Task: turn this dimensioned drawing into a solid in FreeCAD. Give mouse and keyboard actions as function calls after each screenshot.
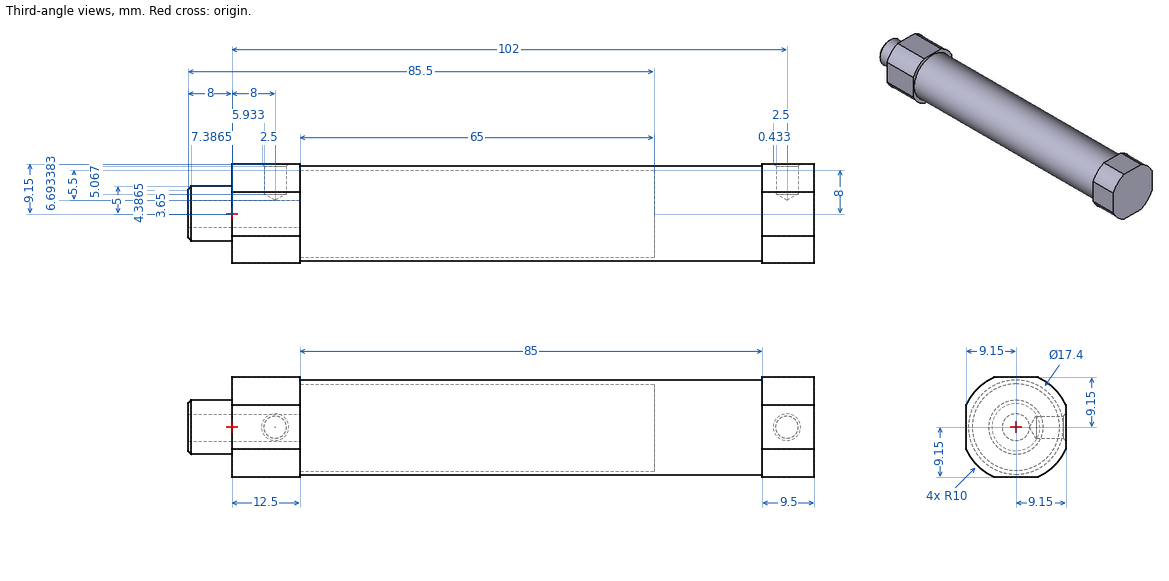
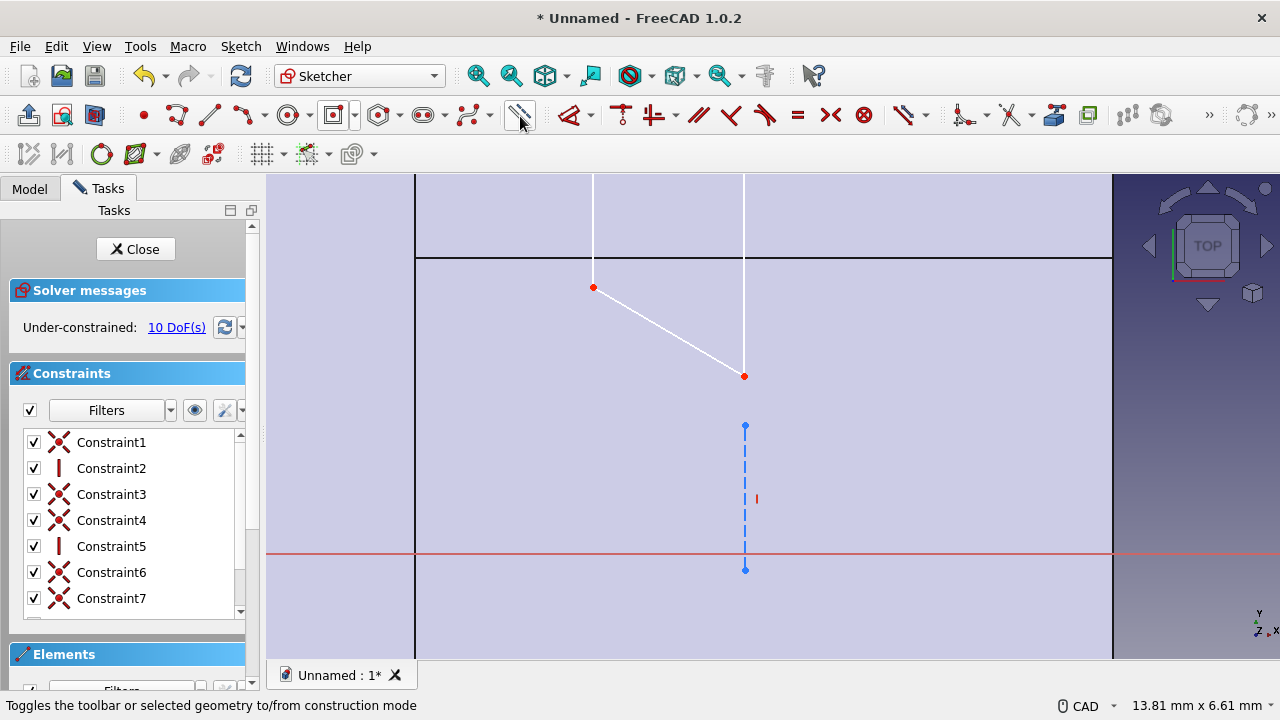
click(568, 116)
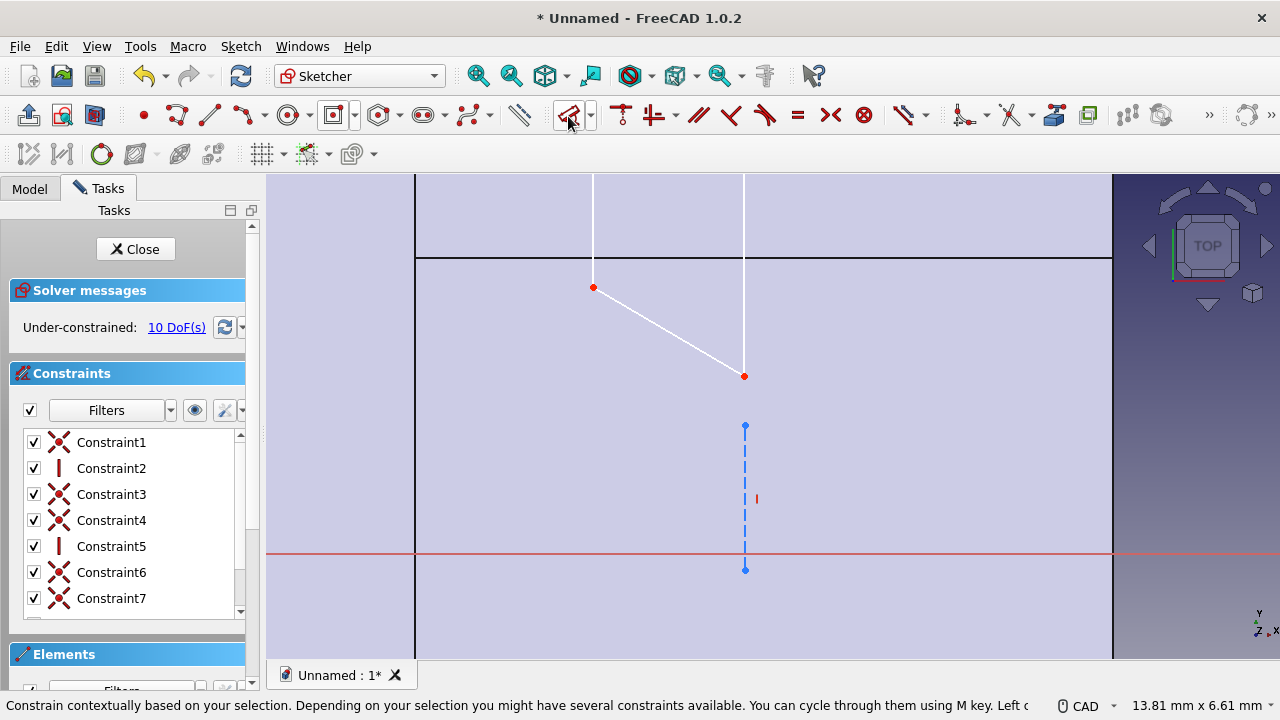
scroll(746, 572, down, 4)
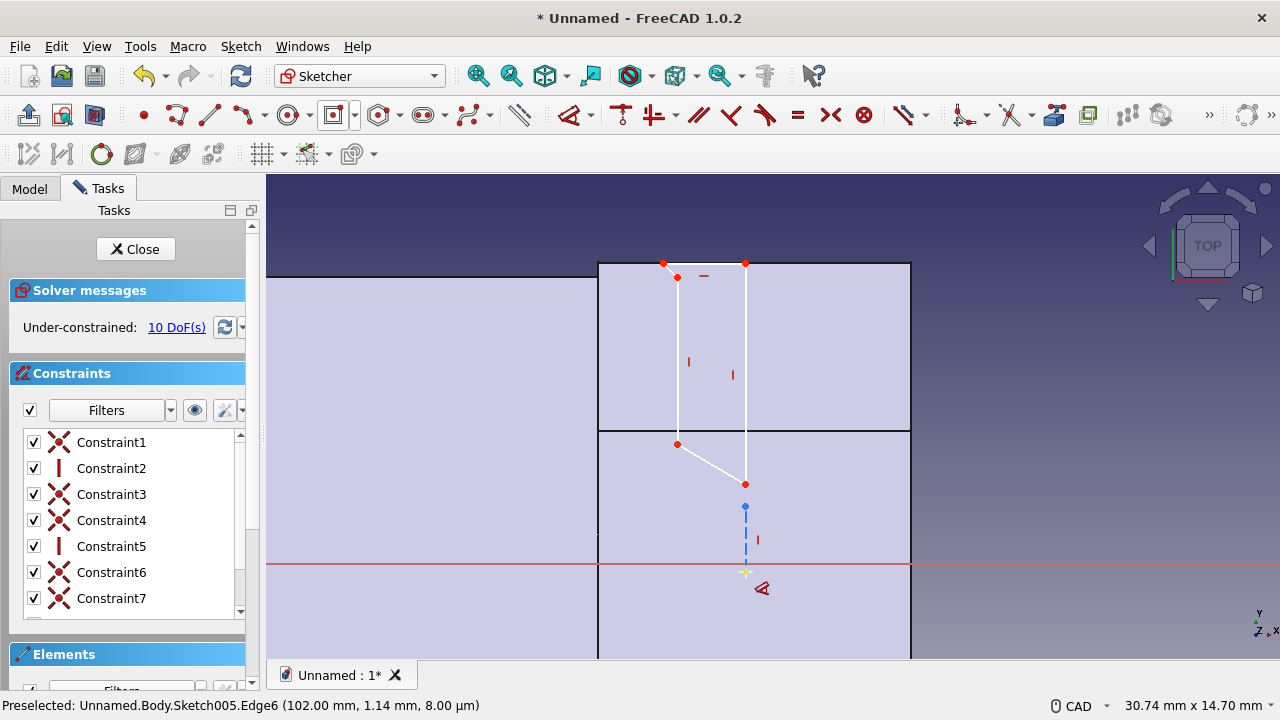
click(721, 264)
click(705, 230)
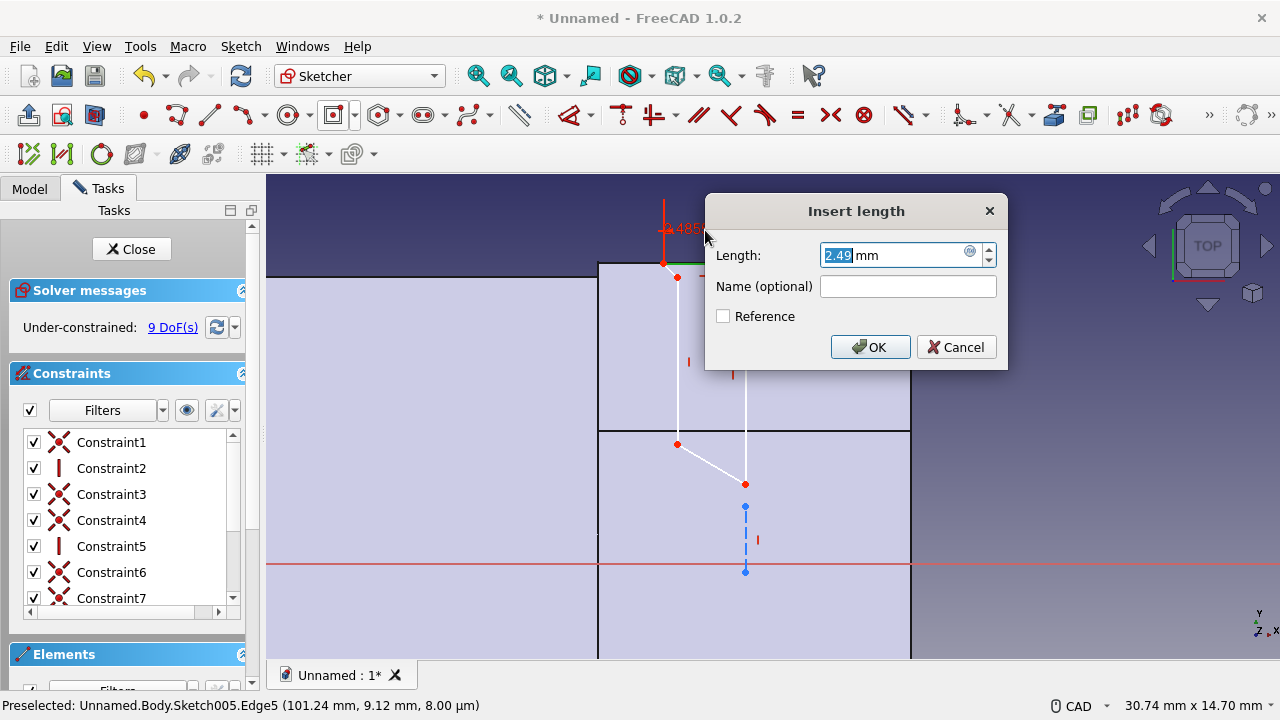
text(2.5)
key(Return)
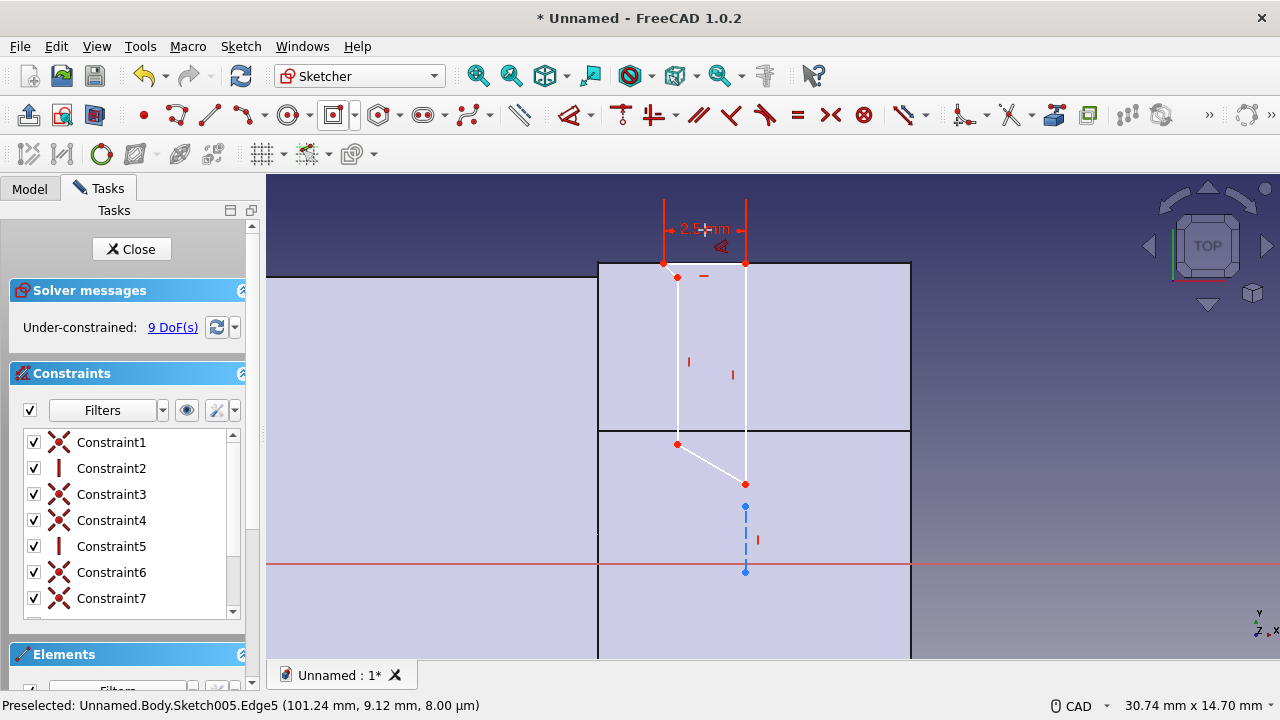
click(746, 485)
click(520, 598)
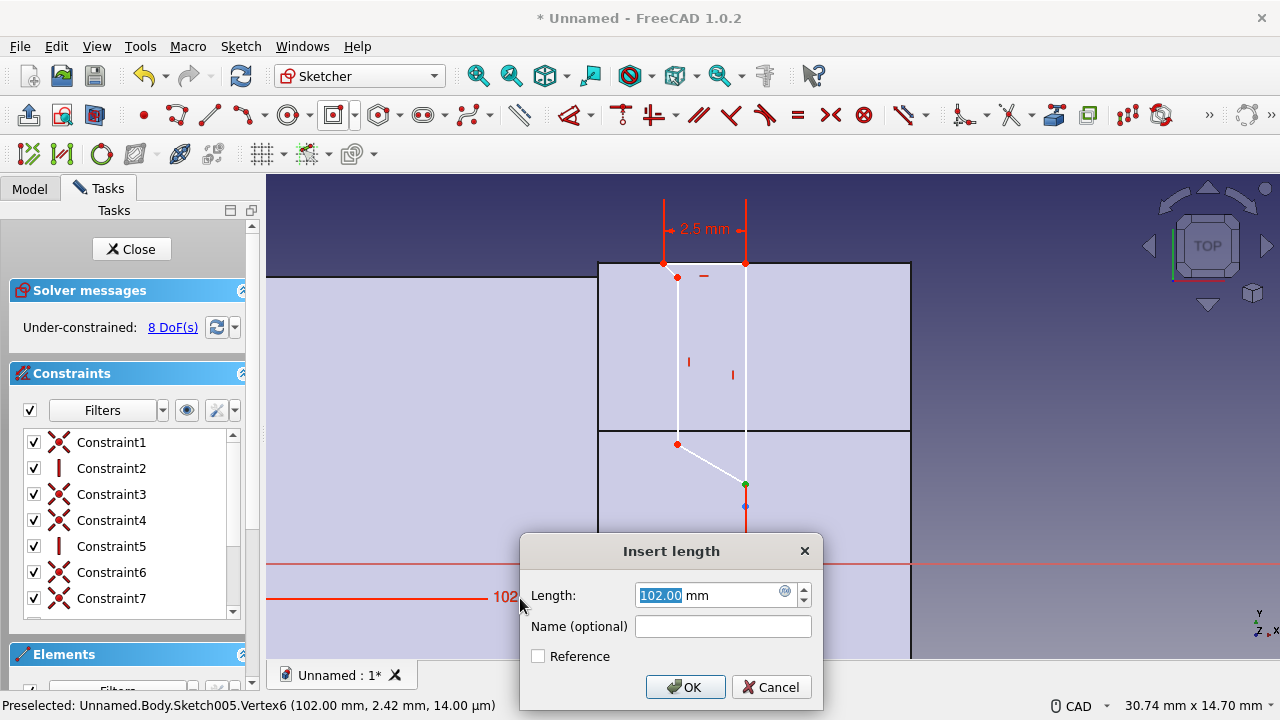
text(102)
key(Return)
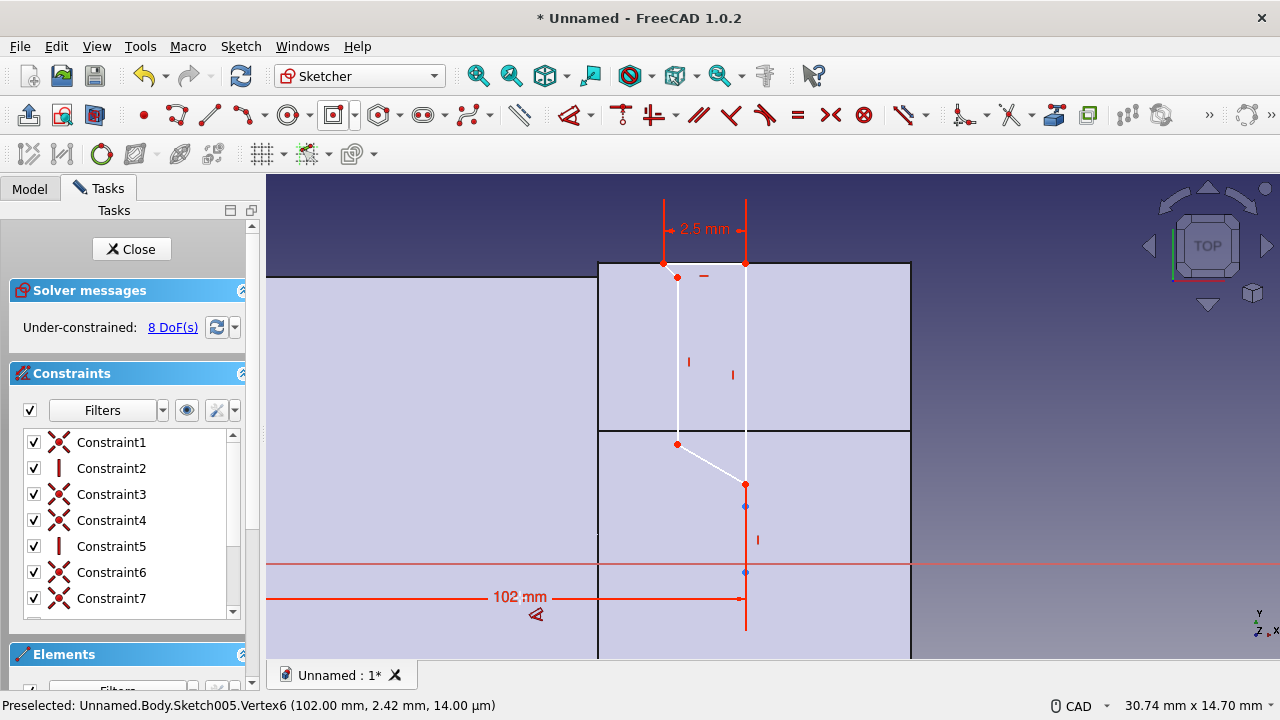
click(746, 507)
click(416, 598)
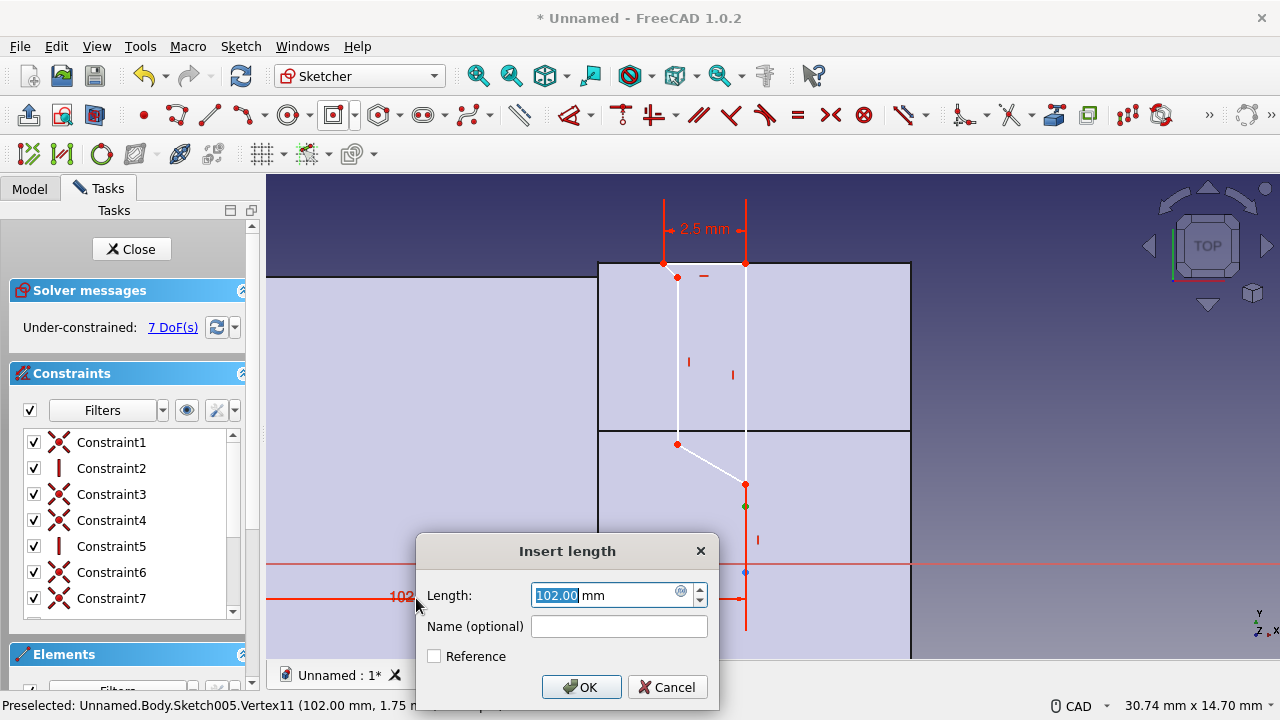
text(102)
key(Return)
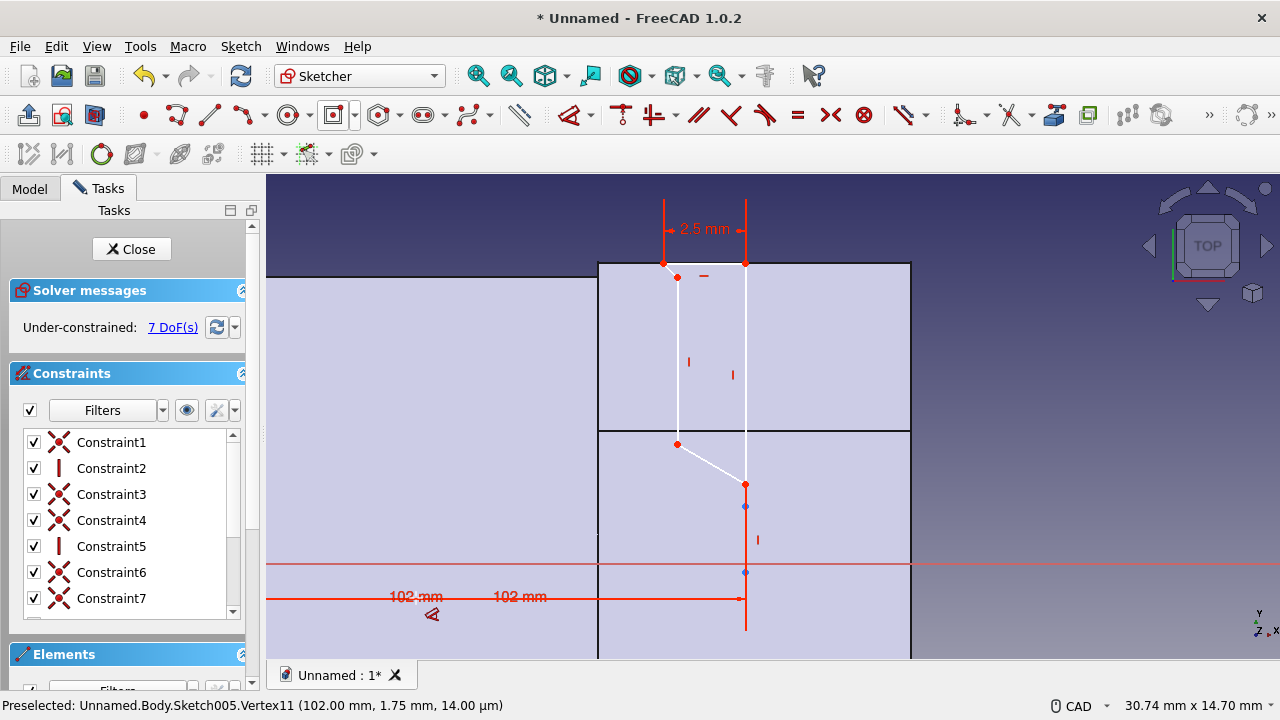
click(678, 328)
click(644, 361)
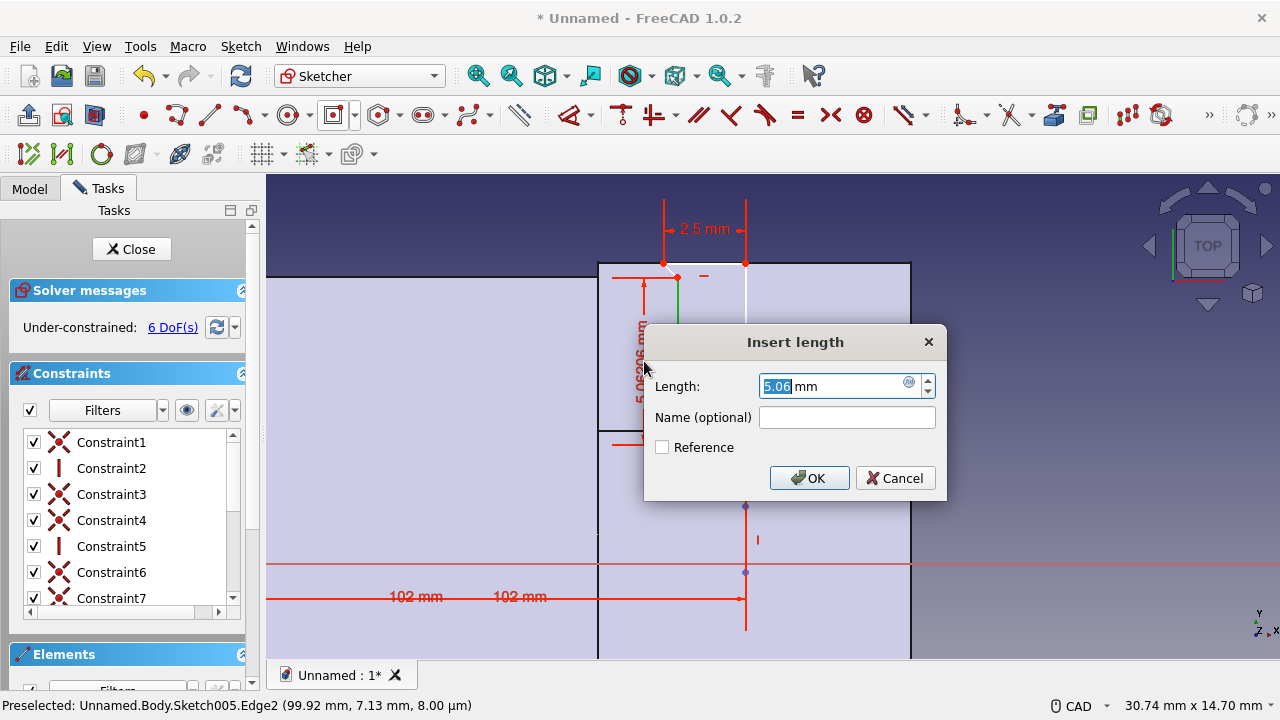
text(5.067)
key(Return)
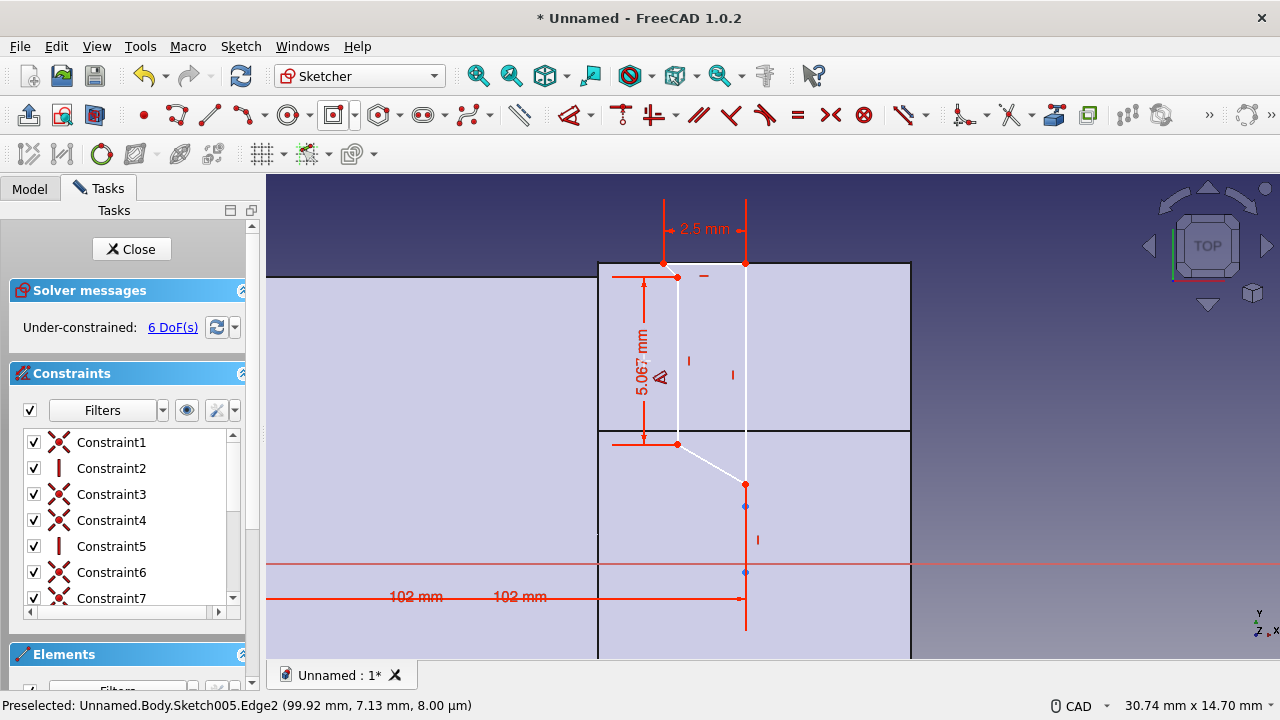
click(664, 264)
click(698, 414)